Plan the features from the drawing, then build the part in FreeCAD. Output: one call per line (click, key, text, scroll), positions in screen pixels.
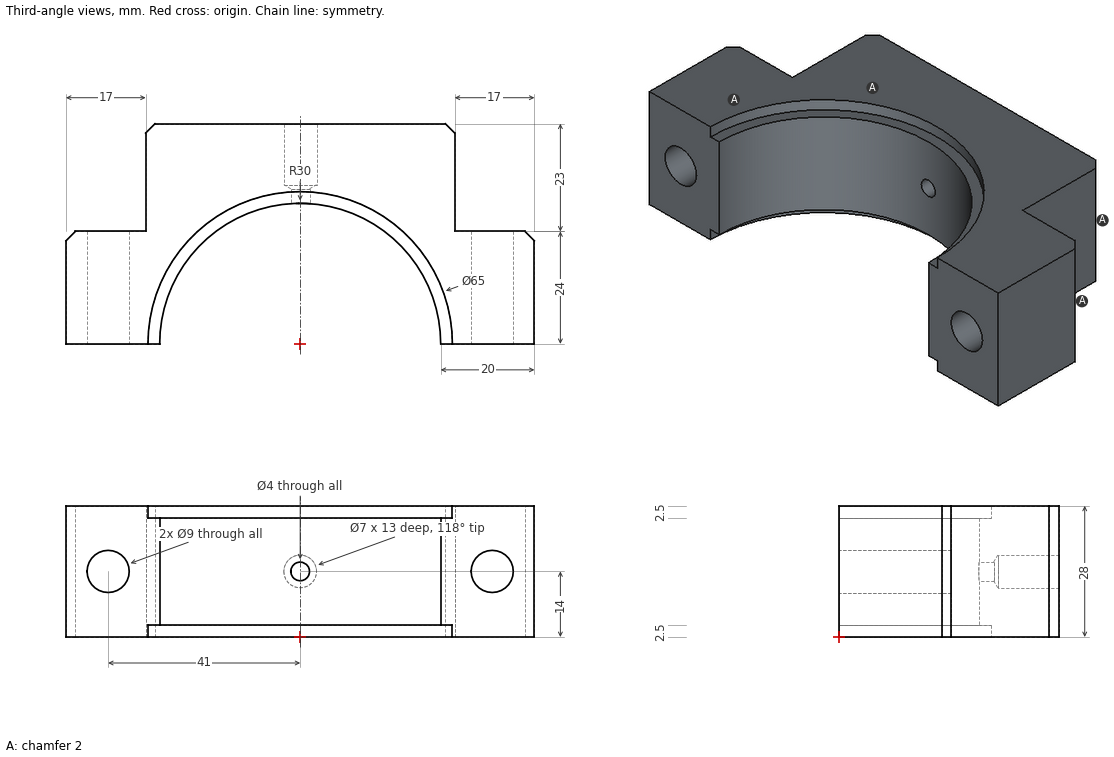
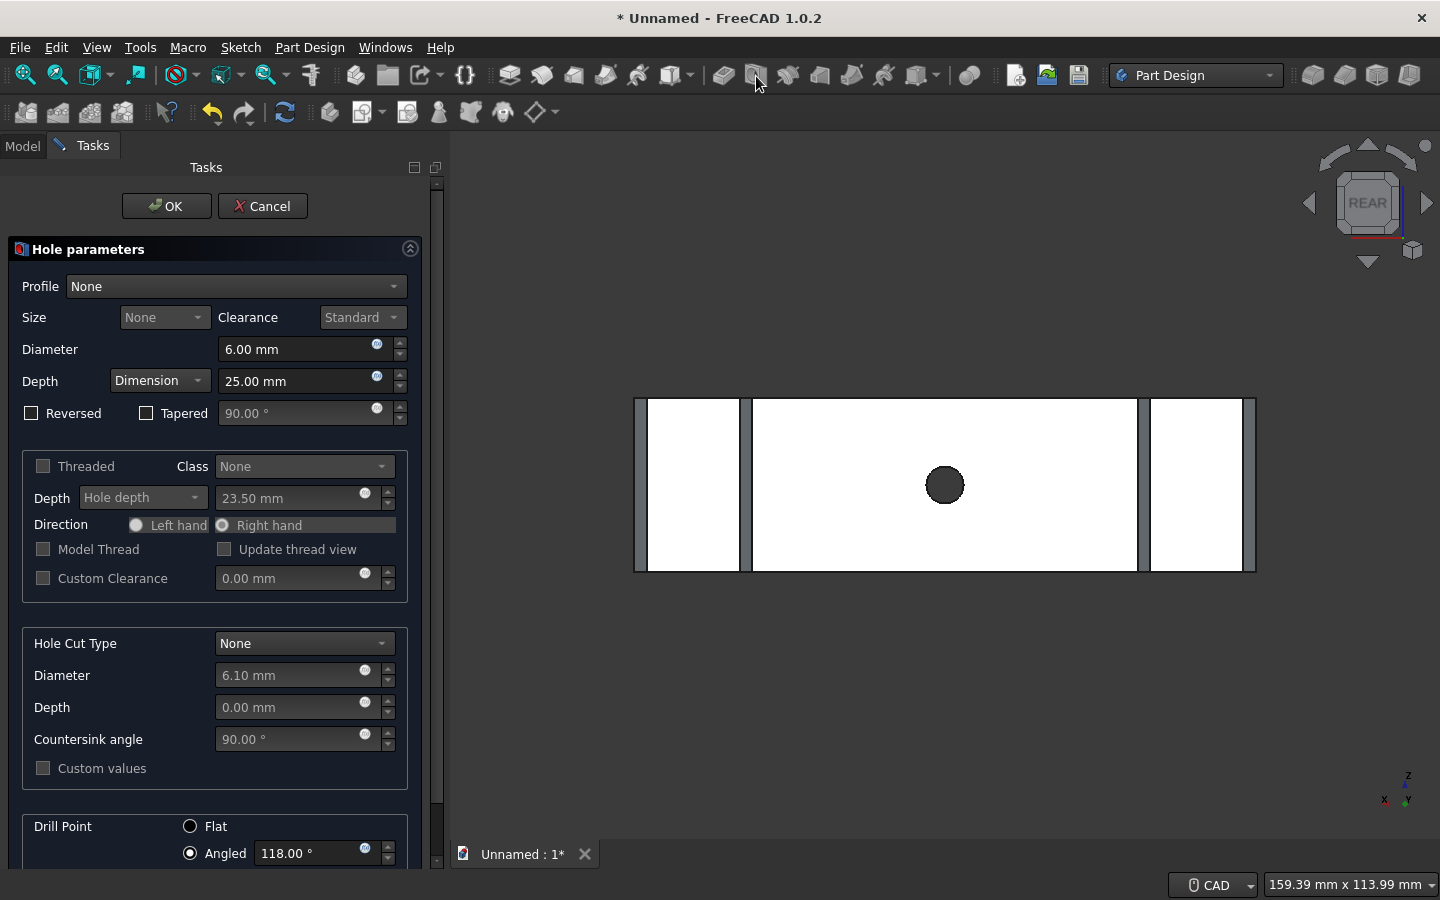
triple_click(305, 349)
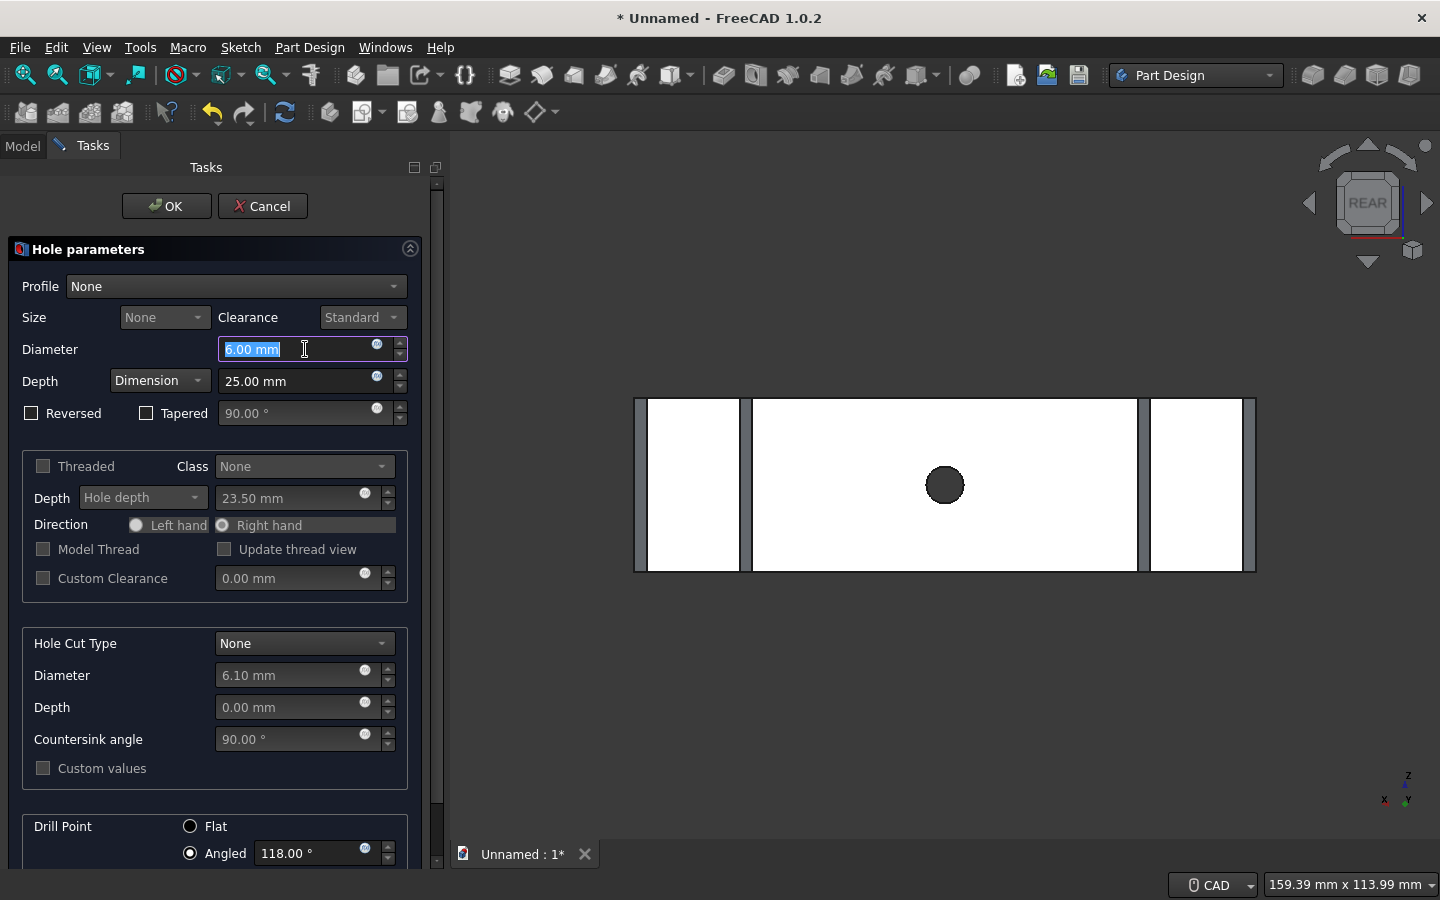
text(7)
key(Tab)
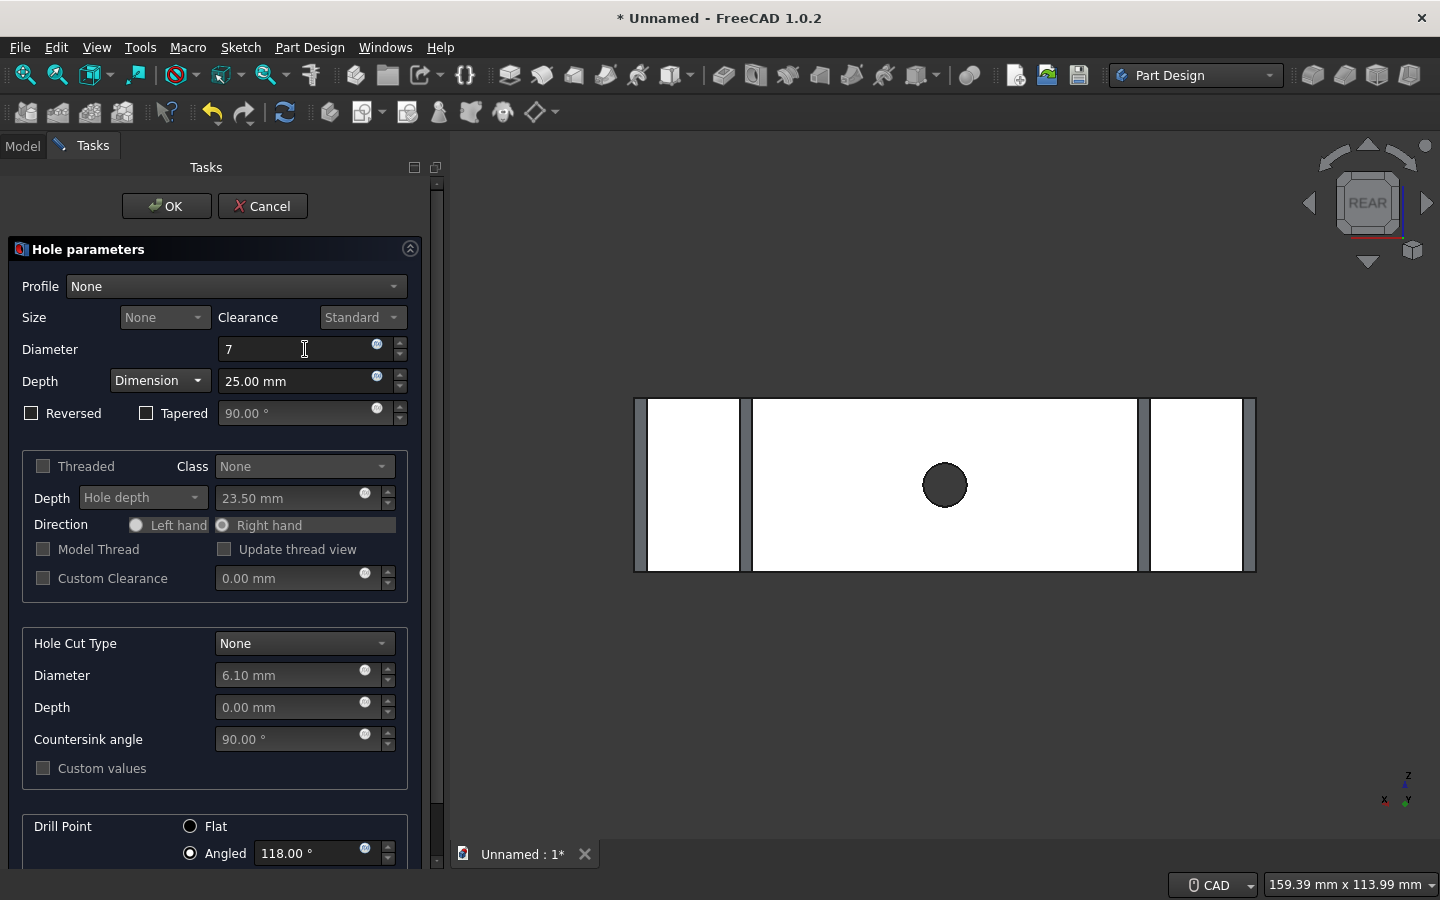
triple_click(305, 381)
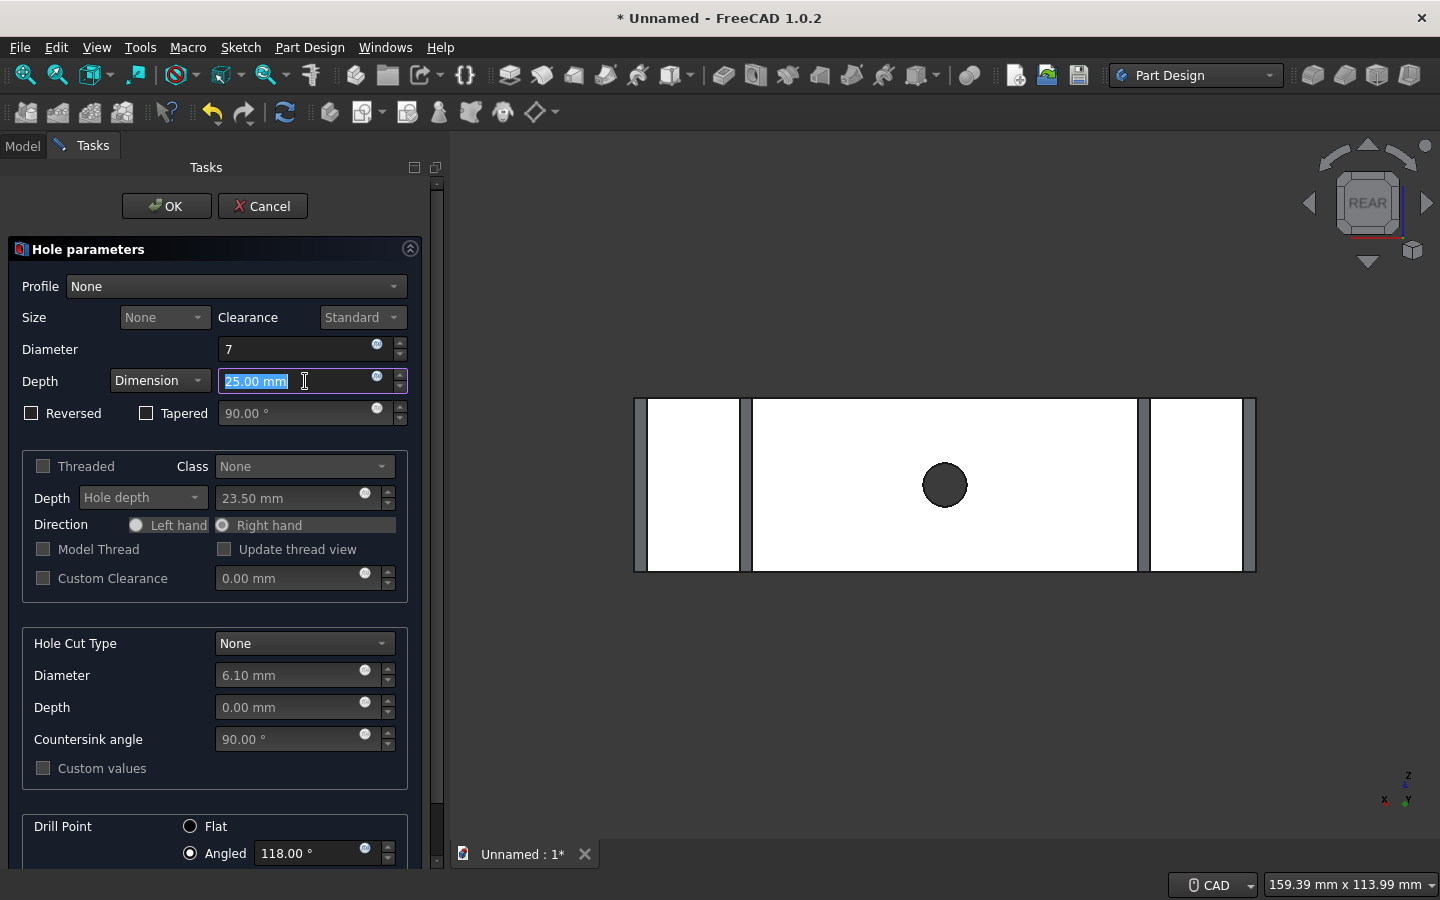
text(13)
key(Tab)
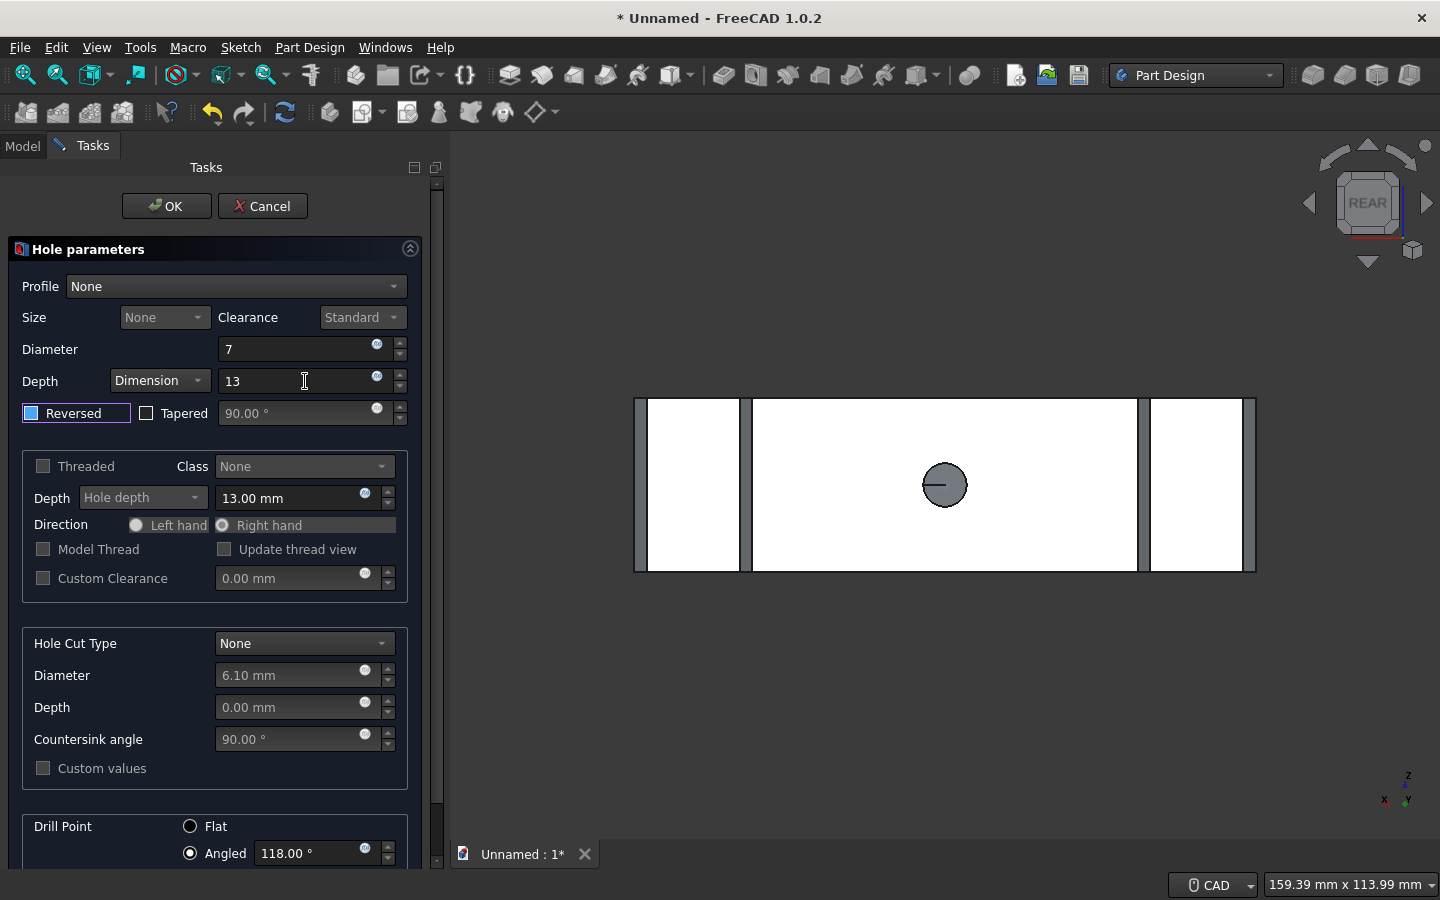
click(167, 206)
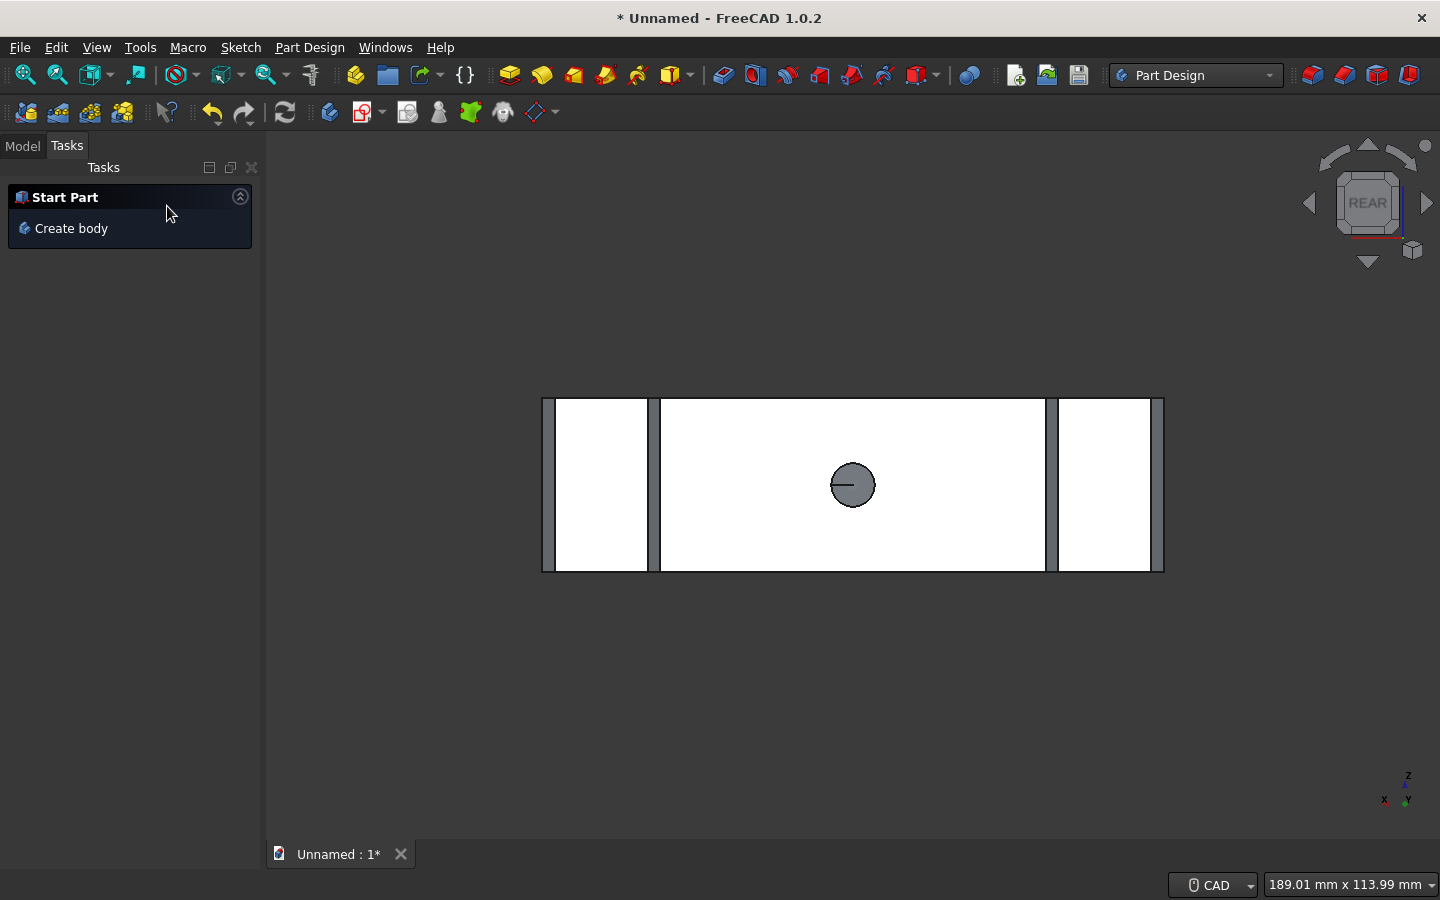
click(601, 459)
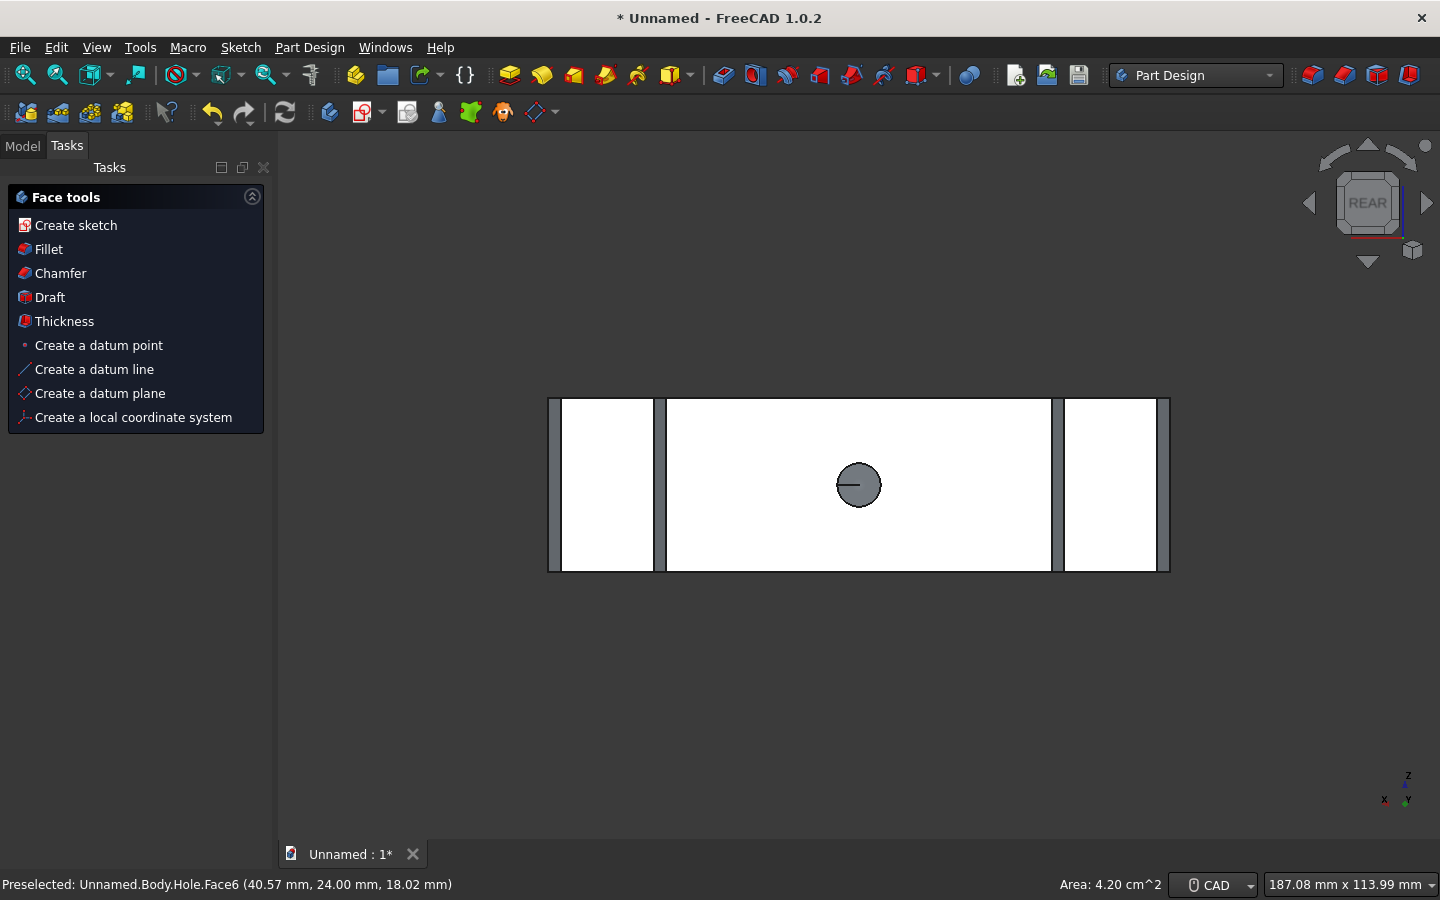
click(362, 112)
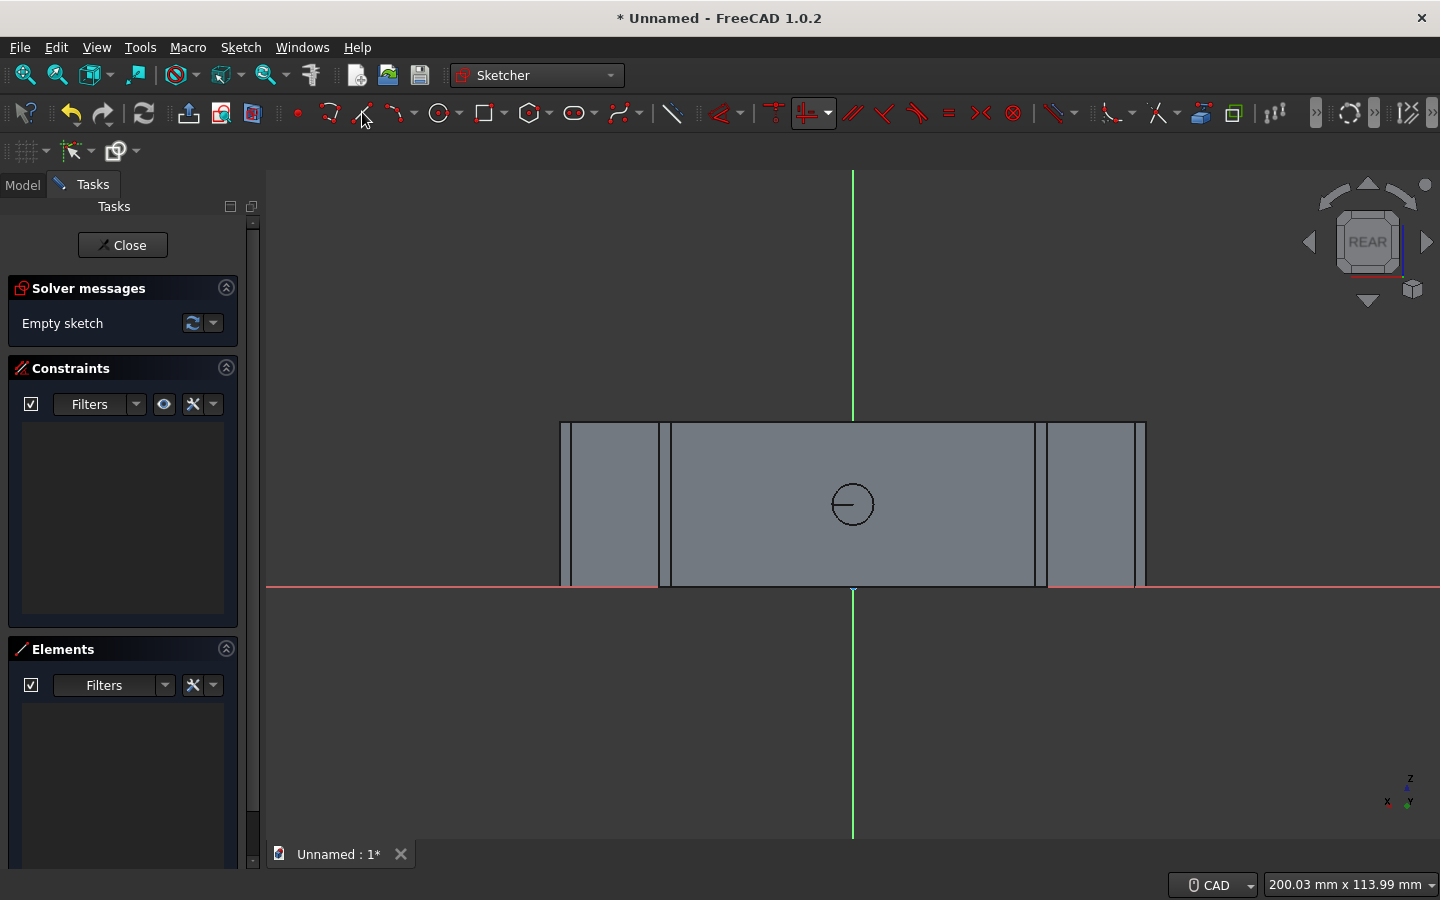
click(440, 114)